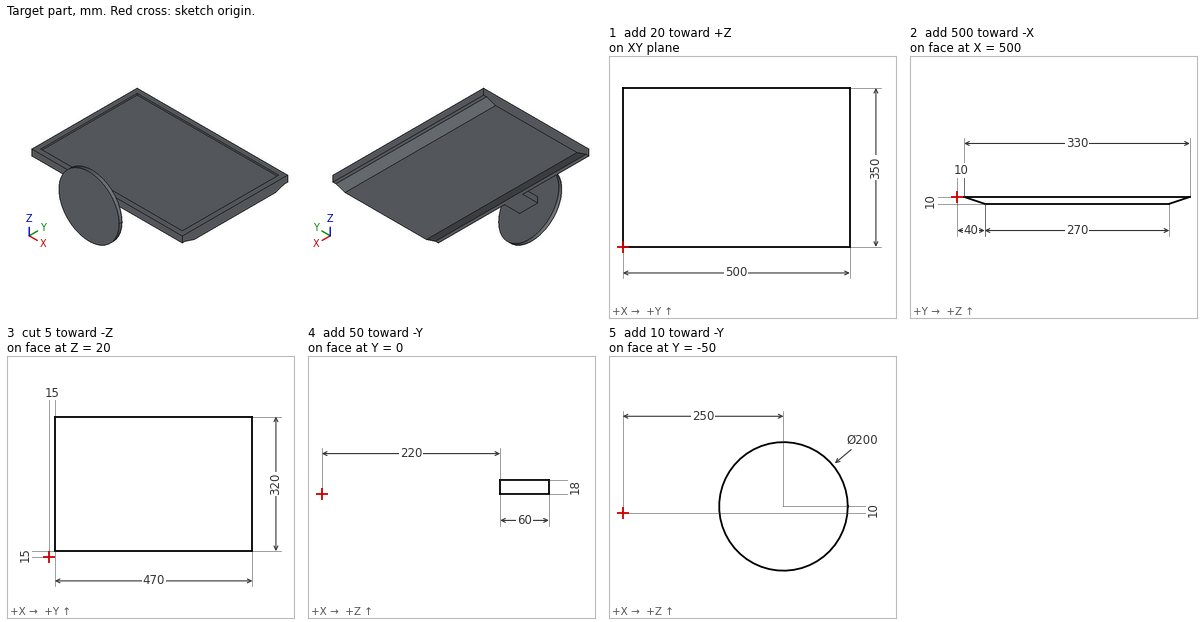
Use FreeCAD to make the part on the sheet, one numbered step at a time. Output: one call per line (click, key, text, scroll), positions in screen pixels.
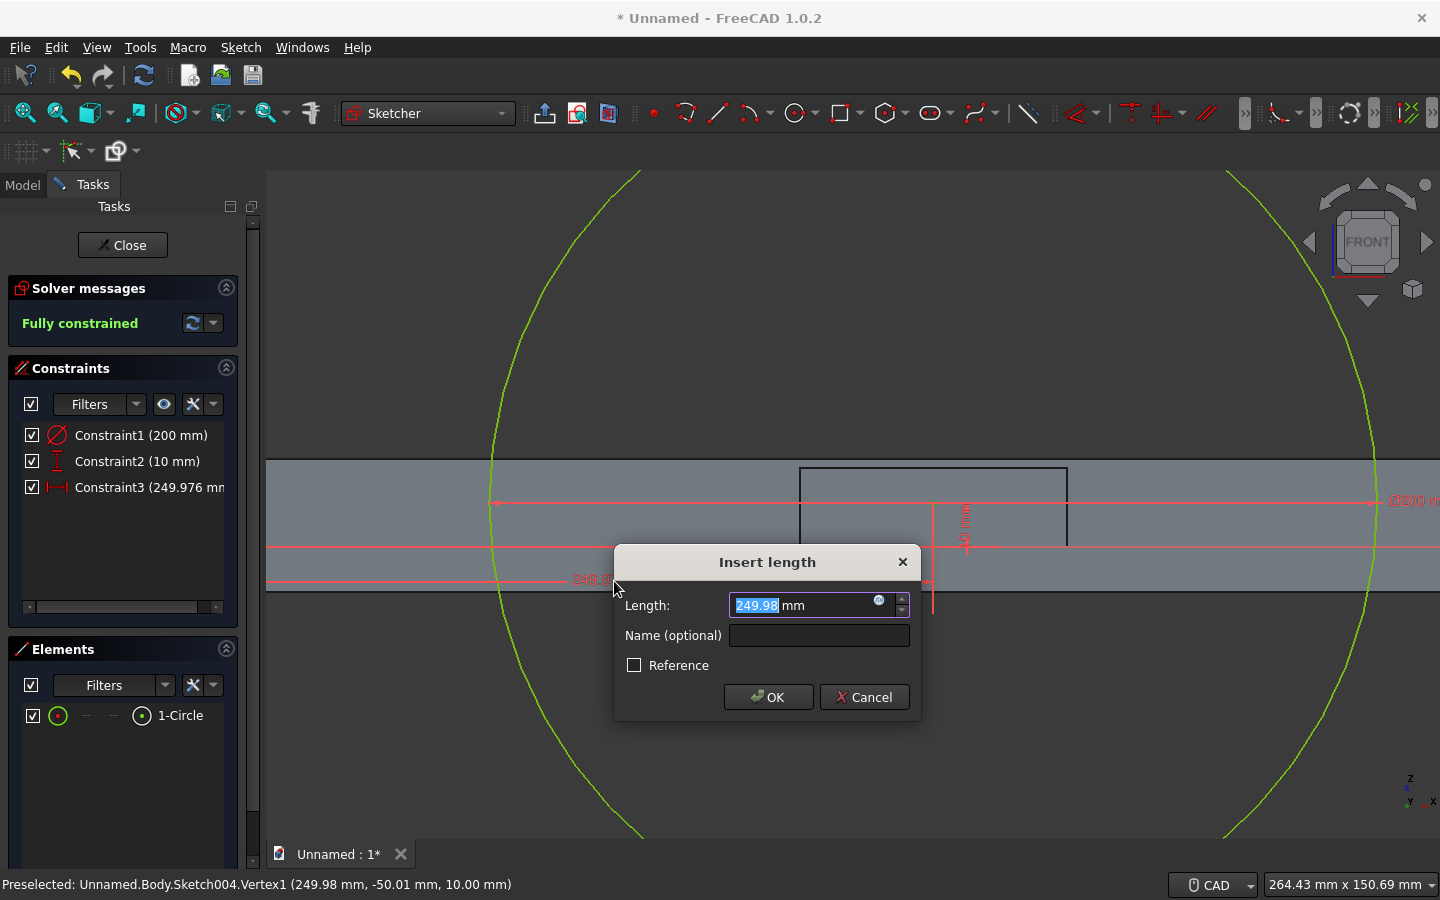
text(250)
key(Return)
key(Escape)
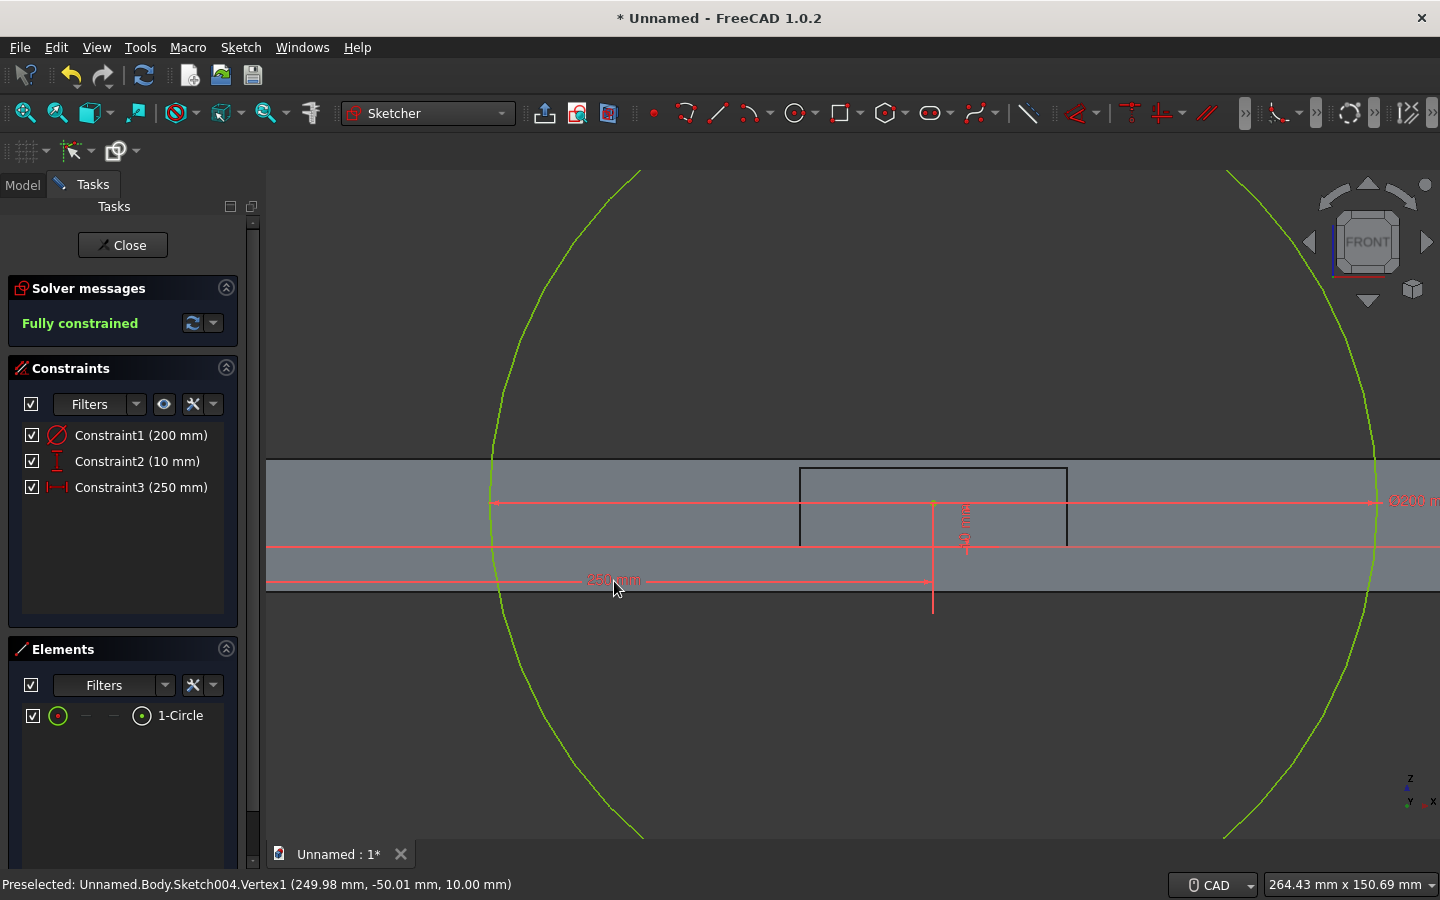
click(123, 245)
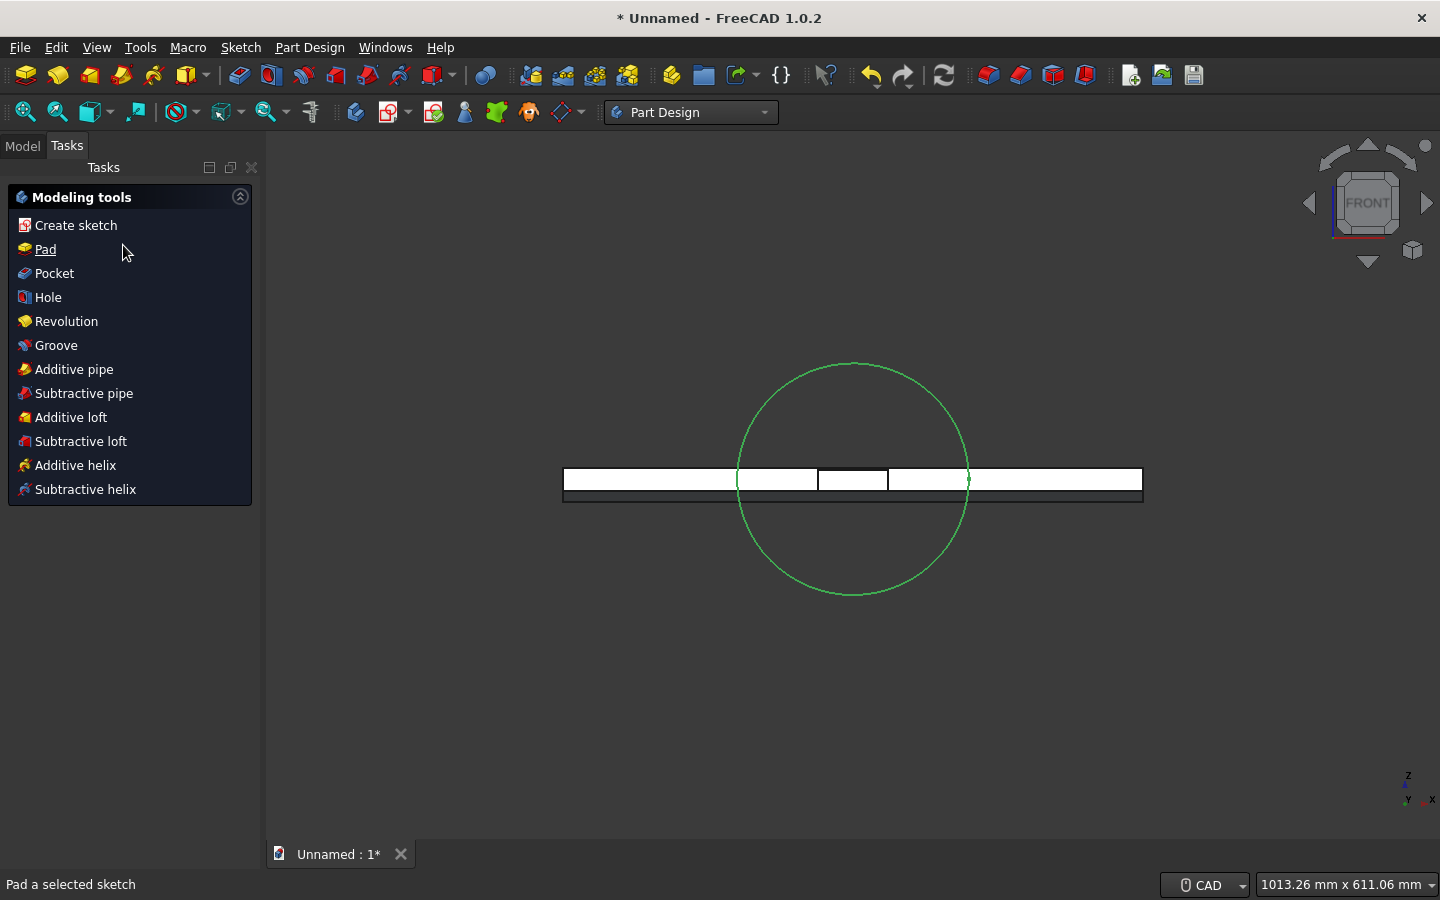
click(26, 76)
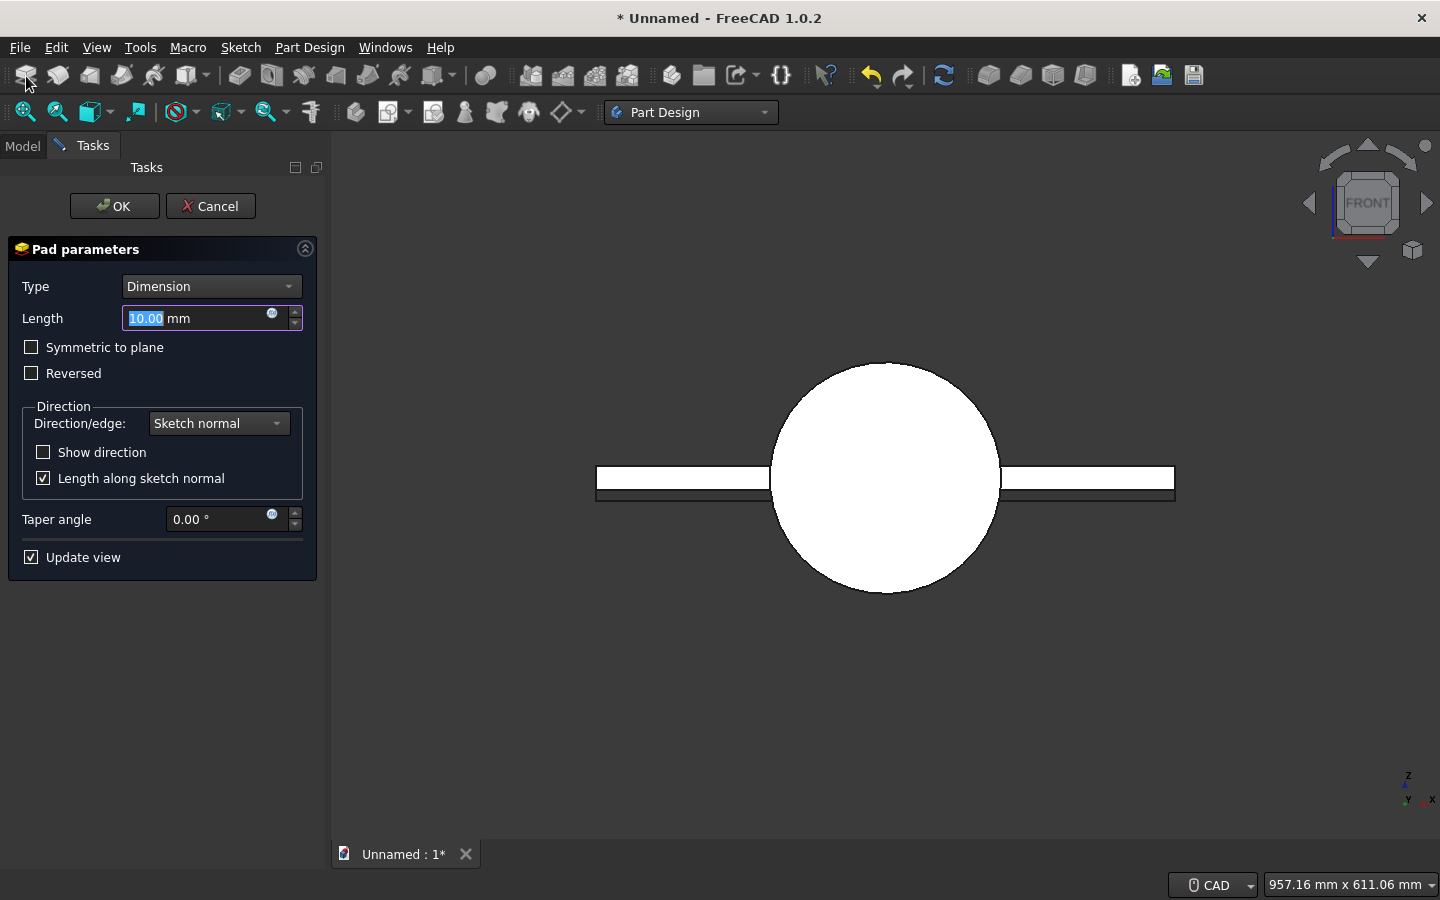
text(10)
key(Tab)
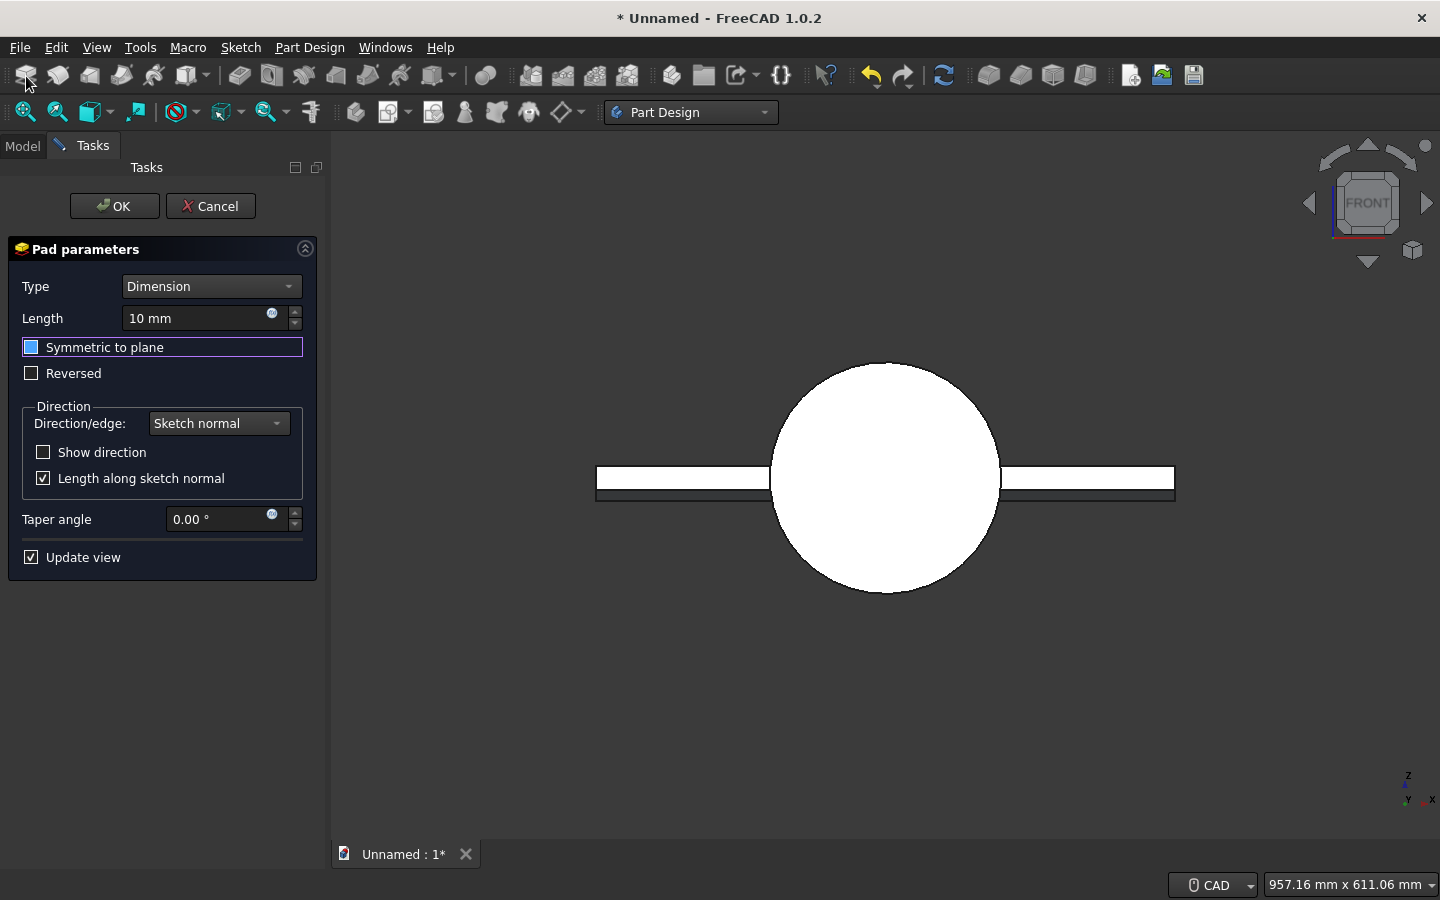
click(115, 206)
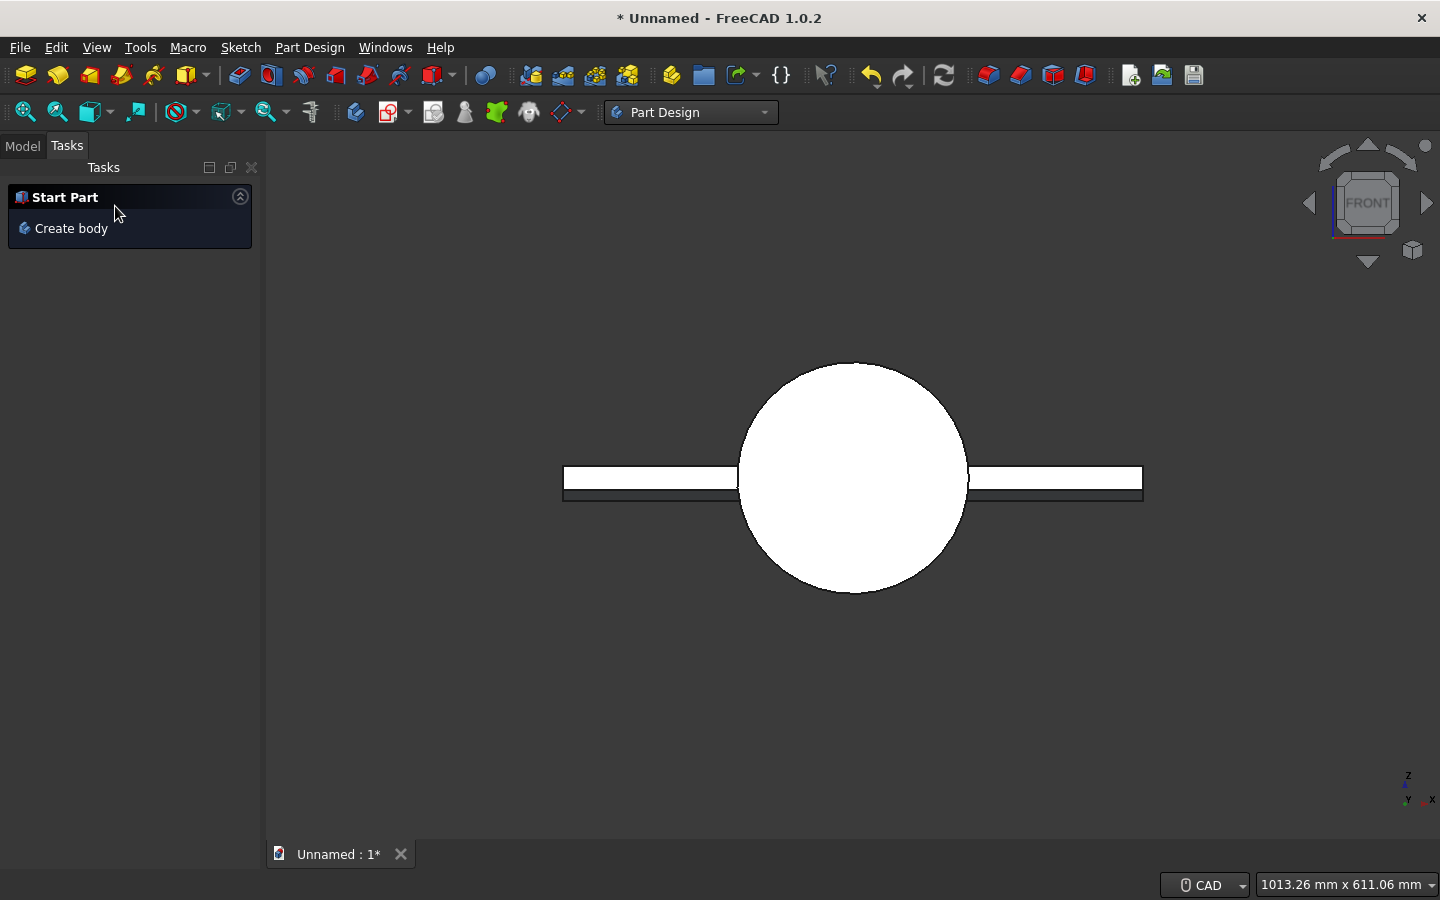
key(0)